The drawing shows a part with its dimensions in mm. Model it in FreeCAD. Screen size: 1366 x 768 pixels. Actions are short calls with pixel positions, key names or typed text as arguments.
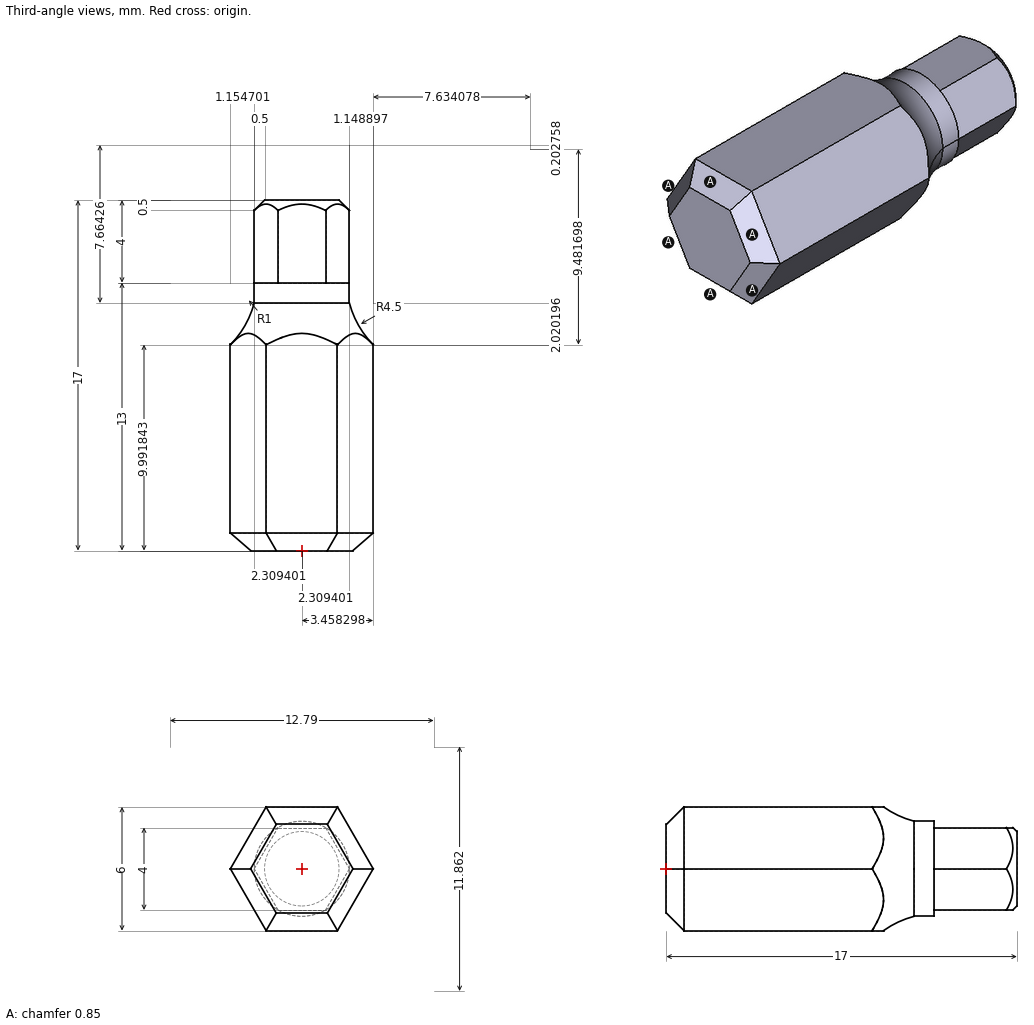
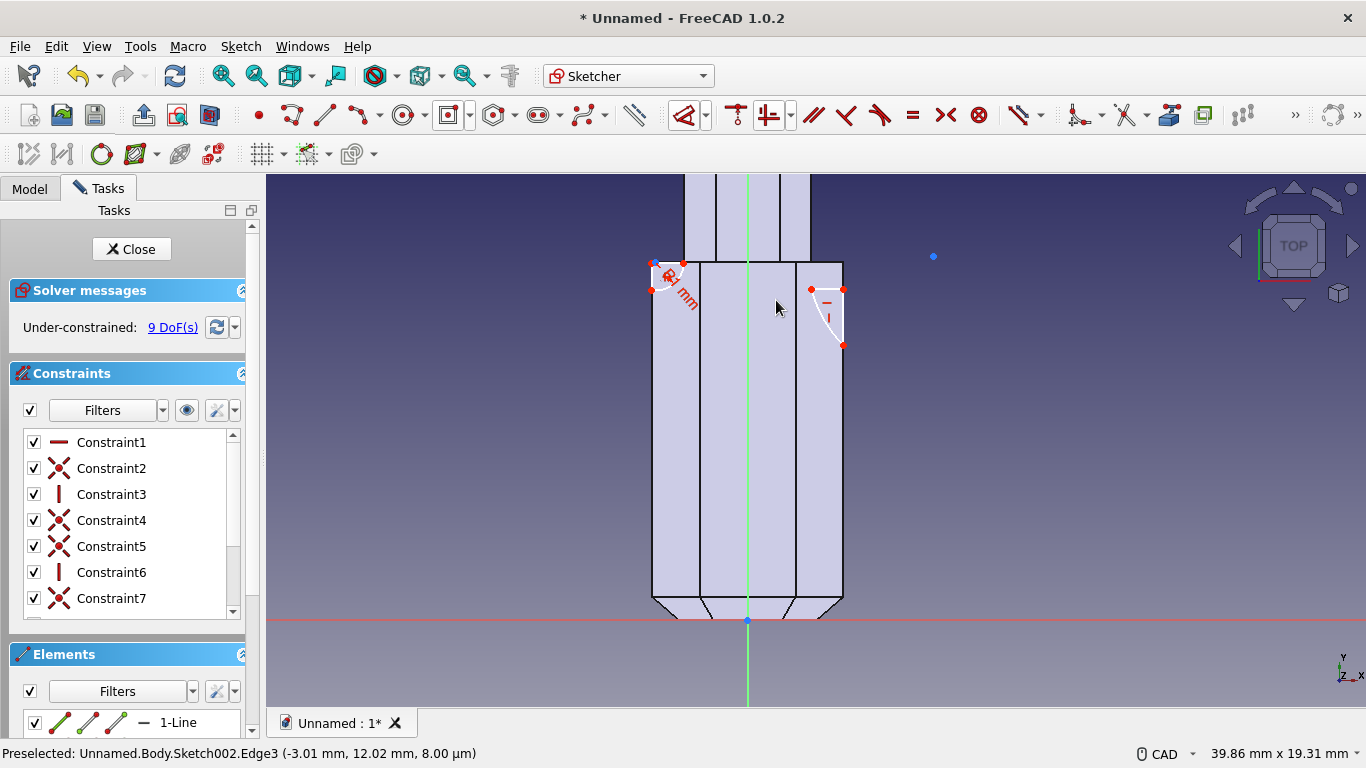
click(818, 308)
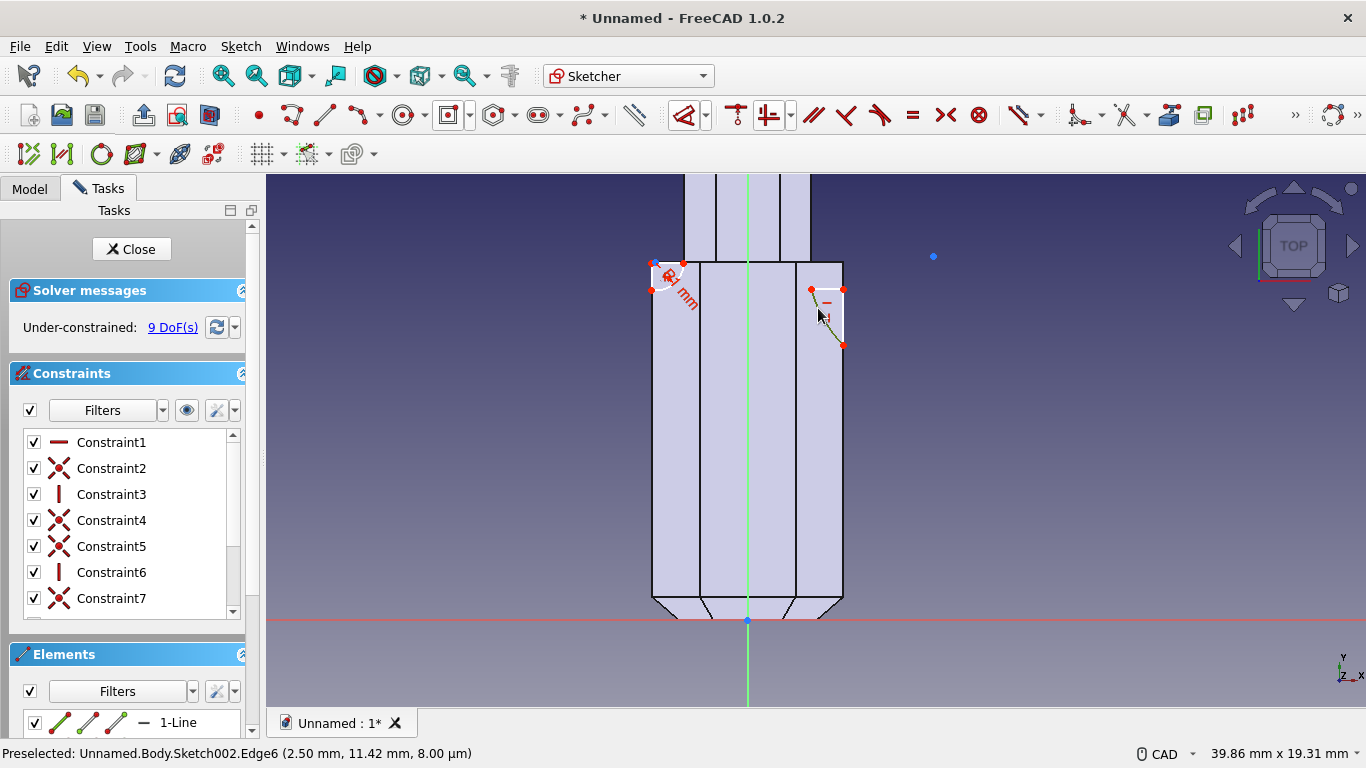
click(706, 116)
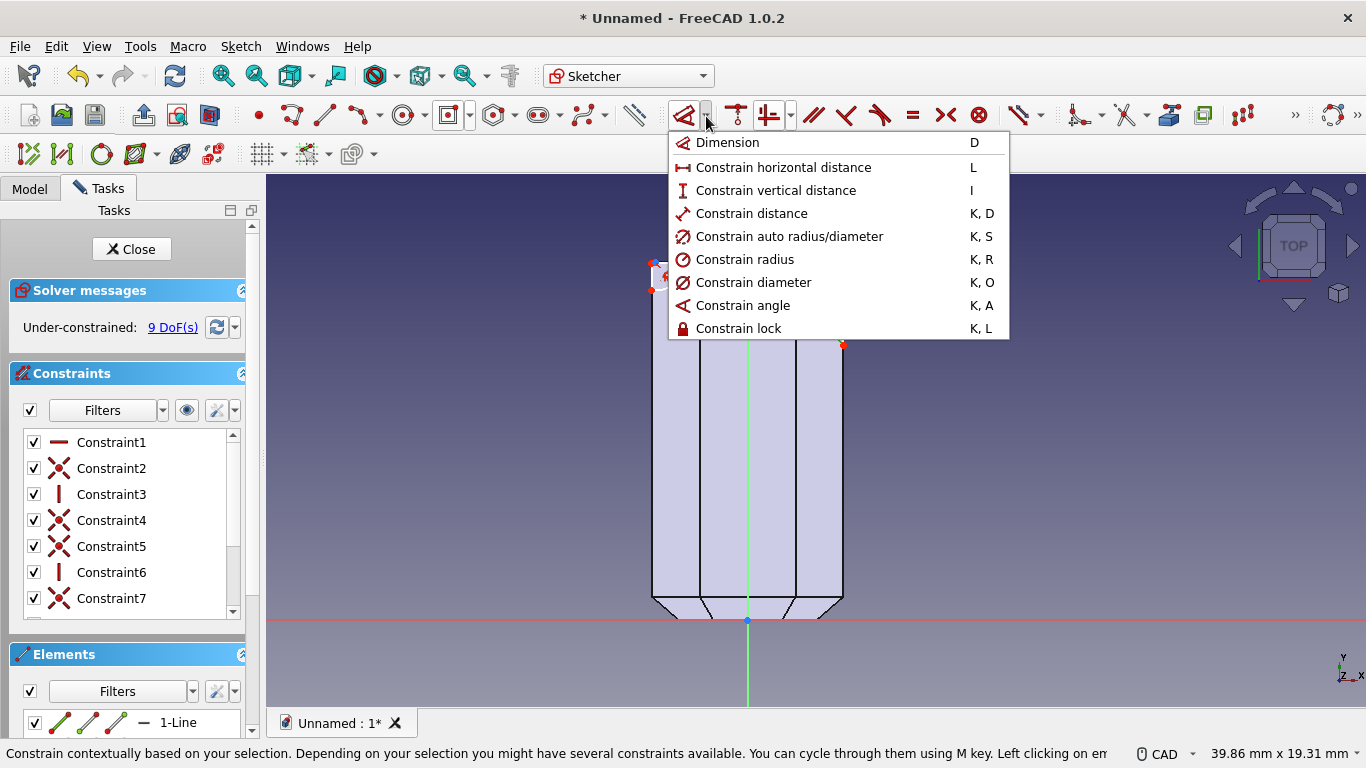
click(839, 260)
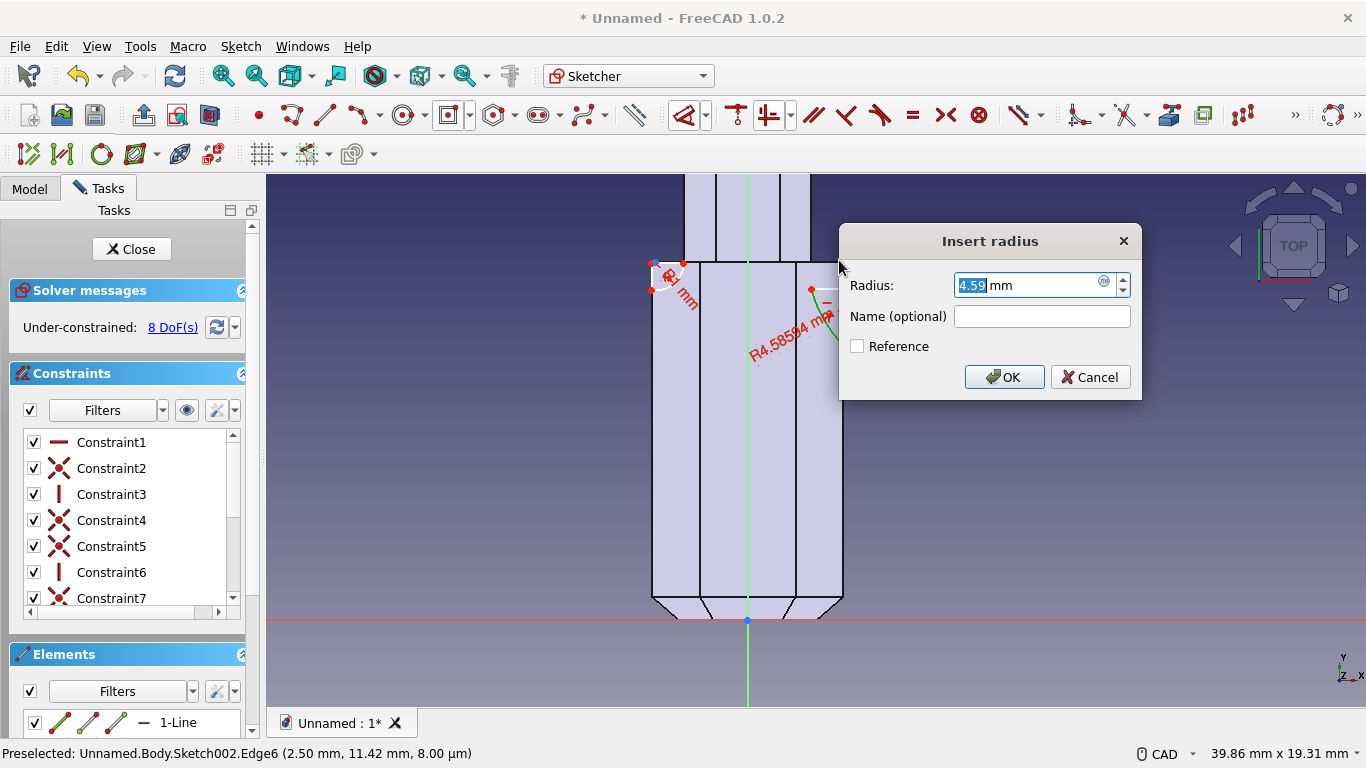
text(4.5)
key(Return)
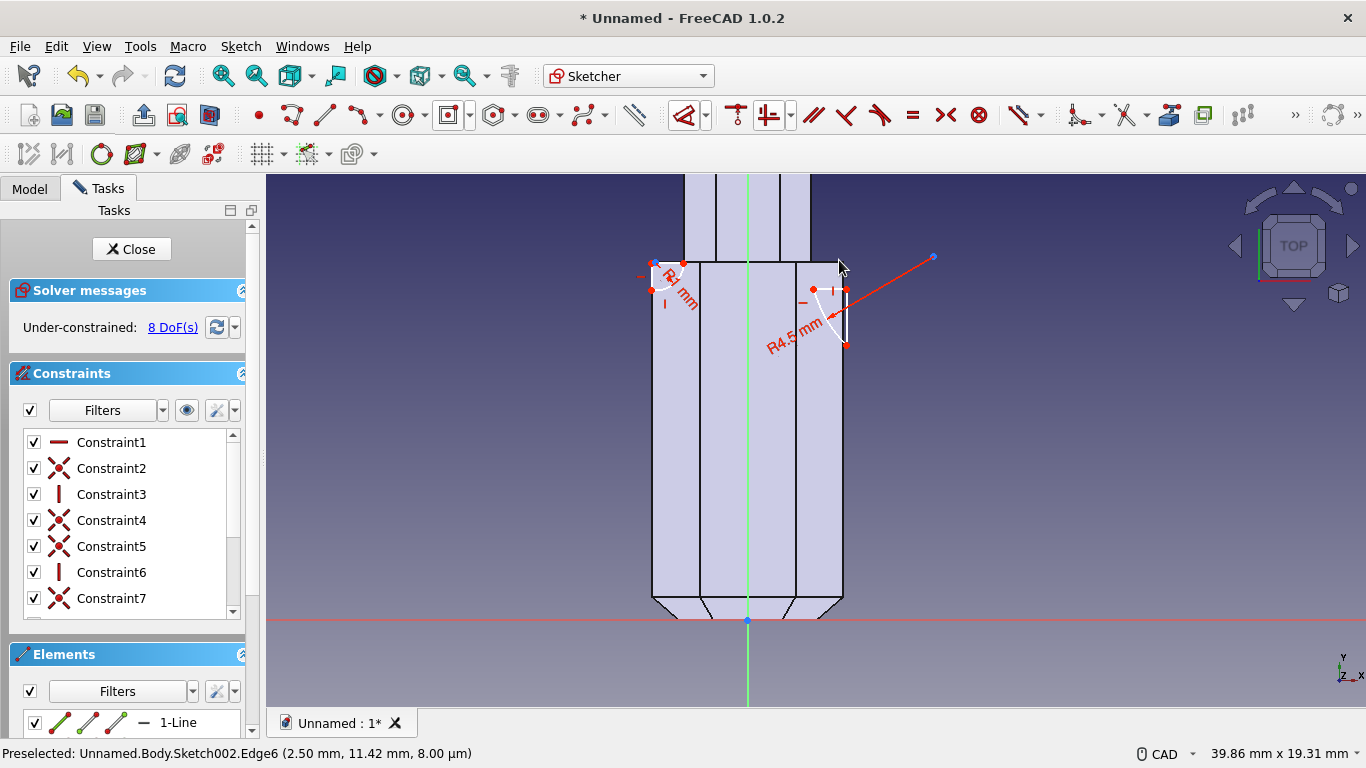
click(684, 263)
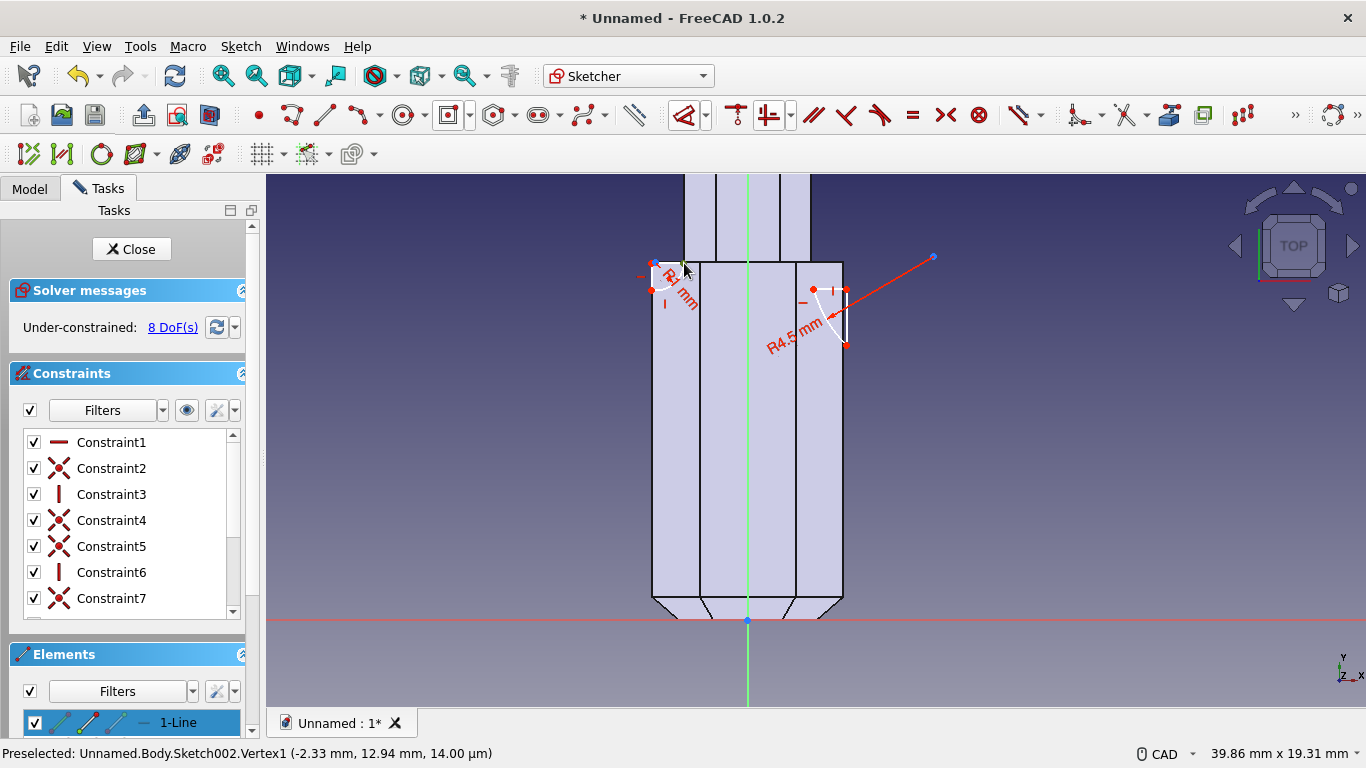
click(706, 116)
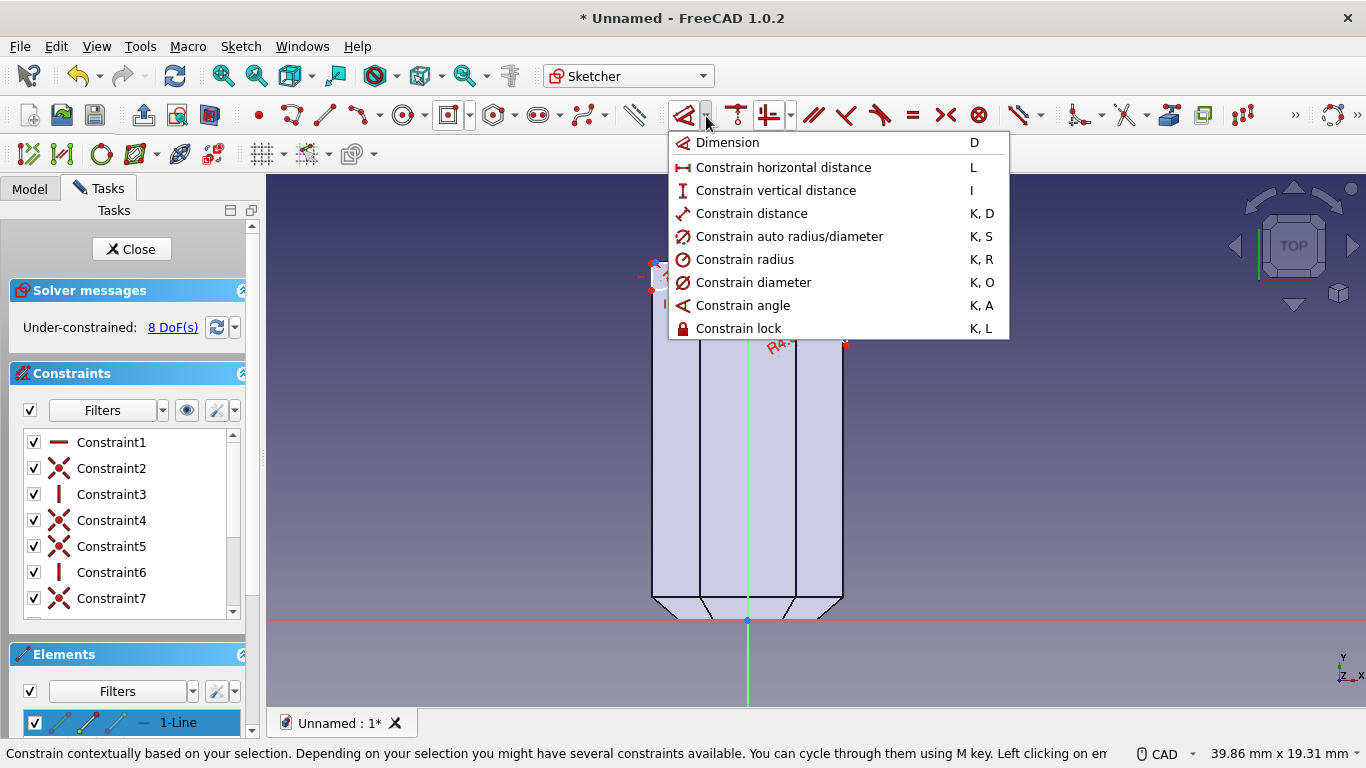
click(839, 190)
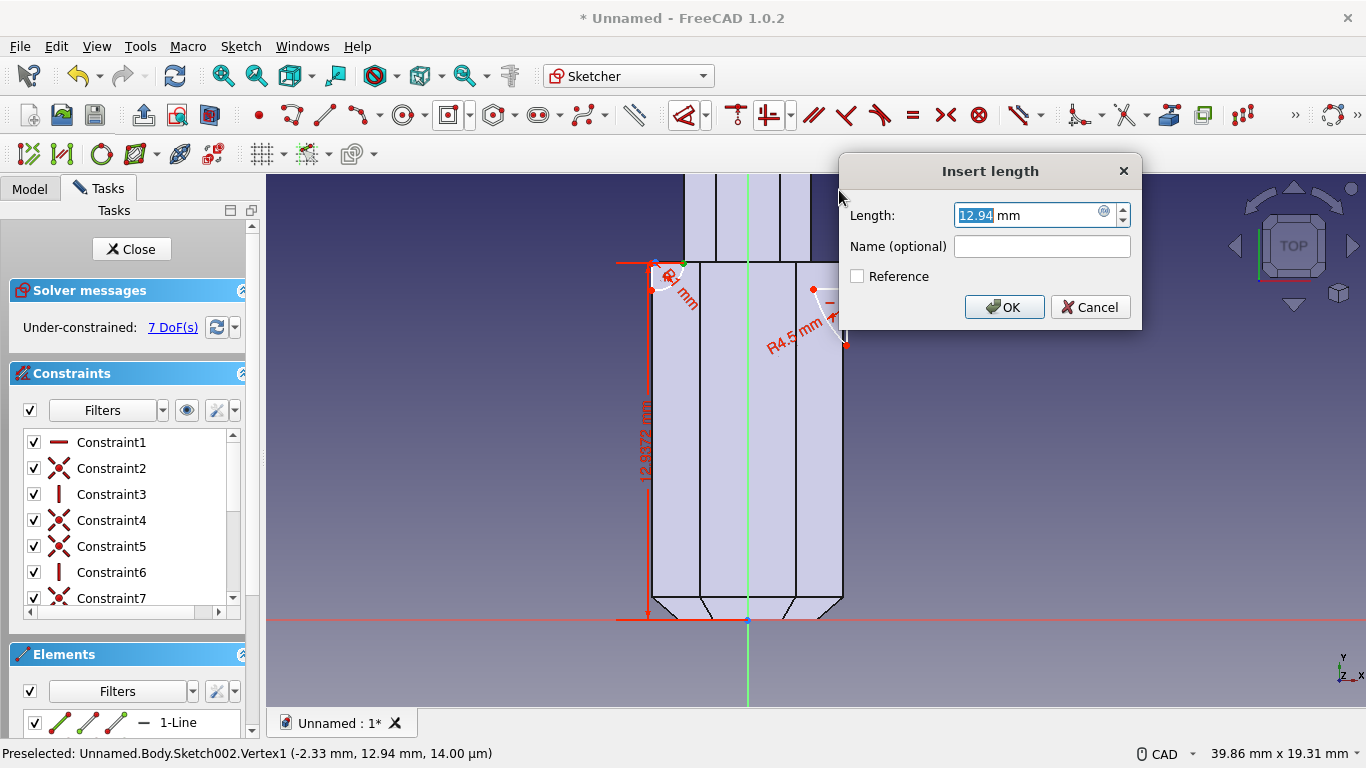
text(13)
key(Return)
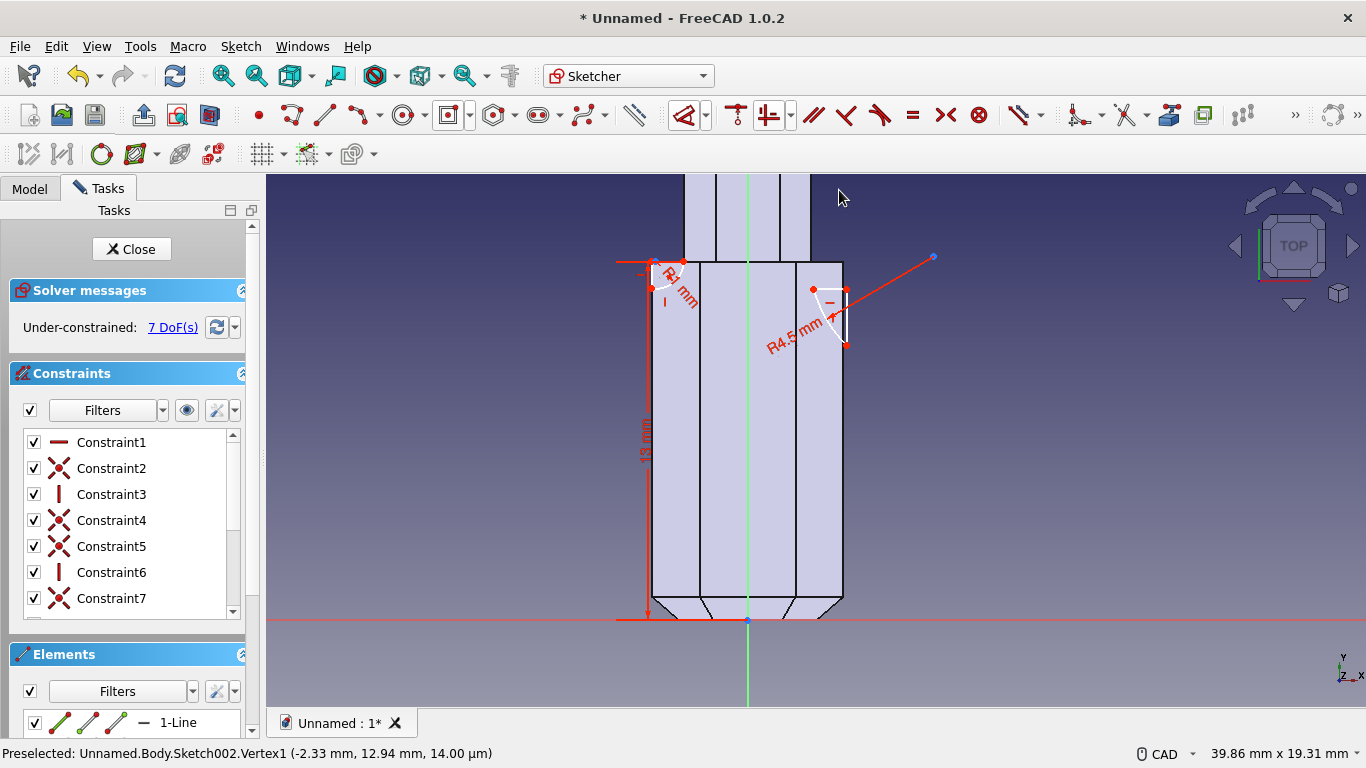
scroll(656, 261, up, 6)